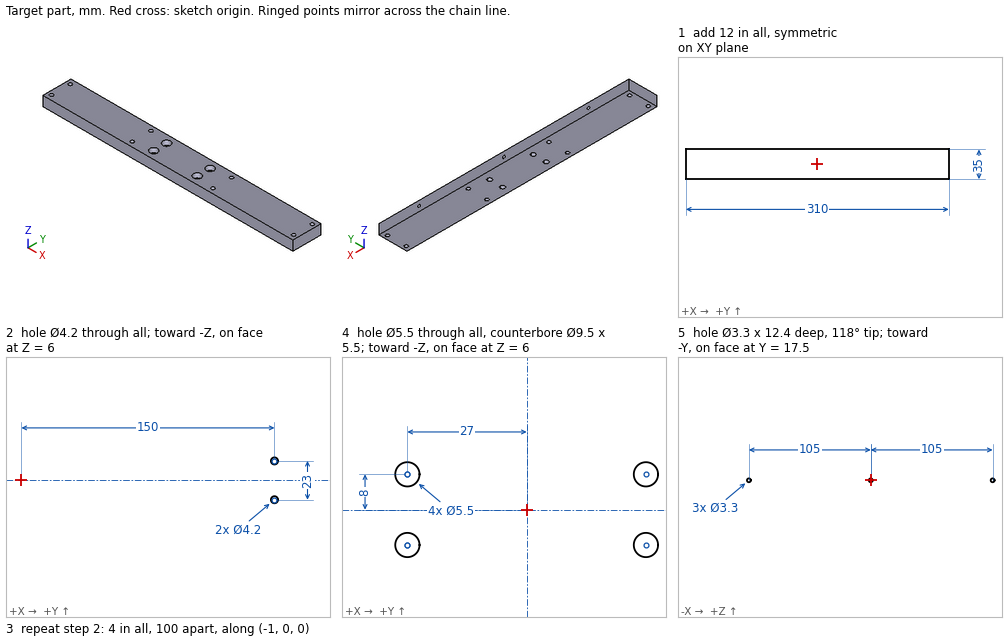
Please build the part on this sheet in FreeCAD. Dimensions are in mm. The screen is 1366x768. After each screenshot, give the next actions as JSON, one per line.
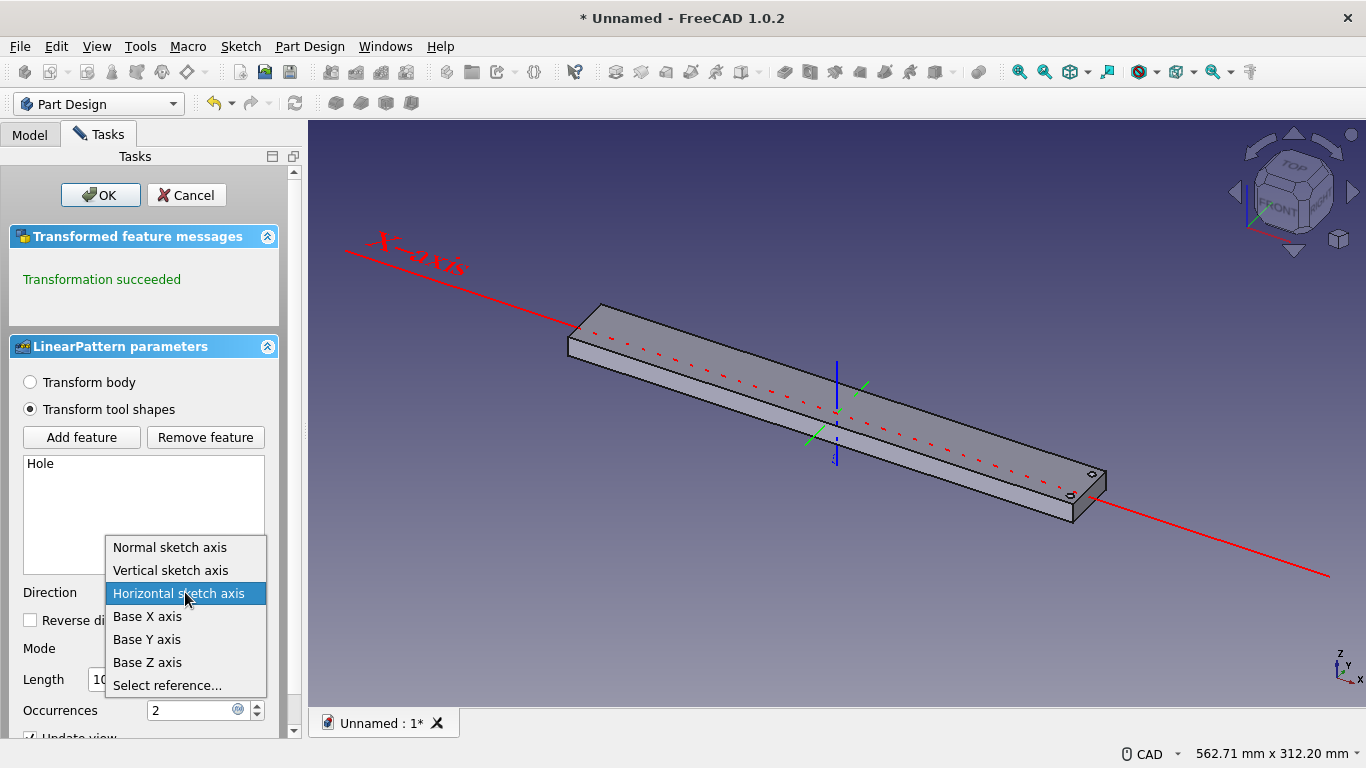
{"action": "left_click", "coordinate": [184, 616]}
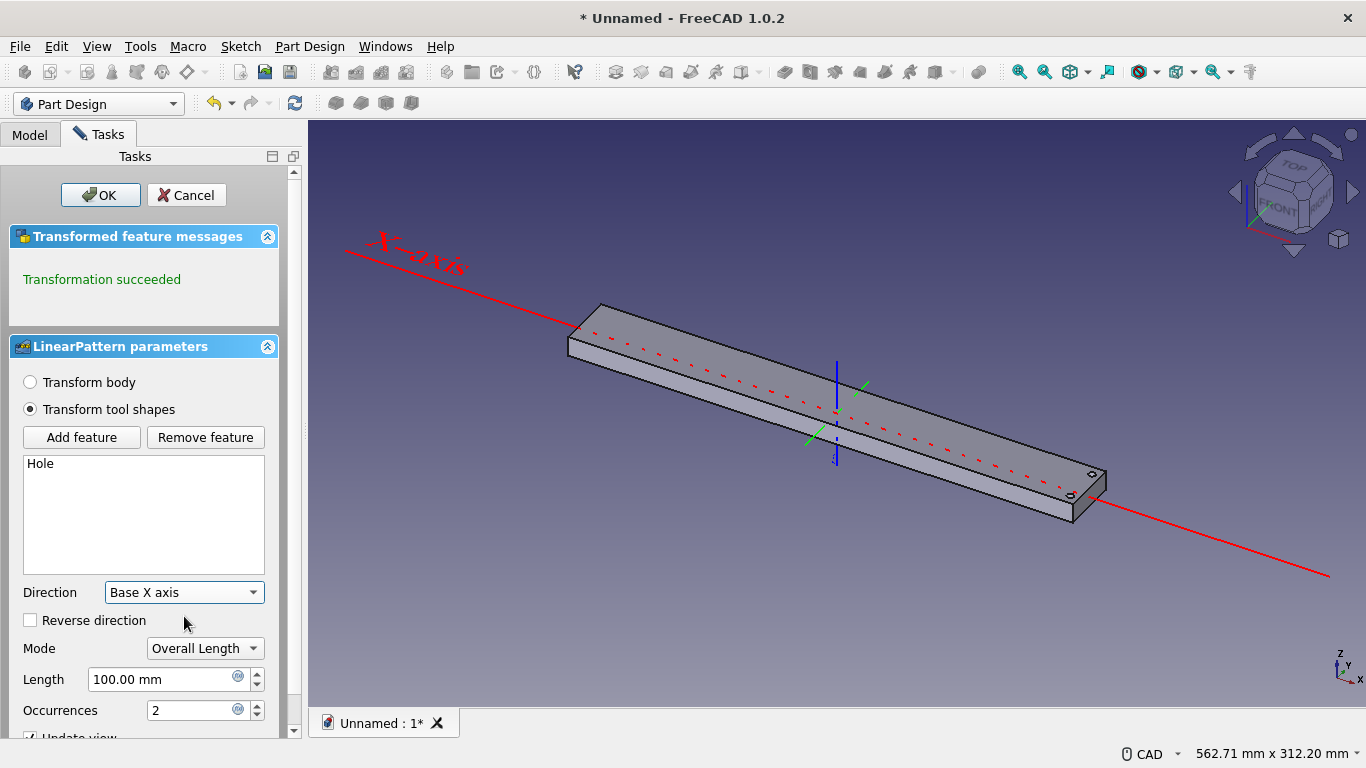
{"action": "left_click", "coordinate": [206, 648]}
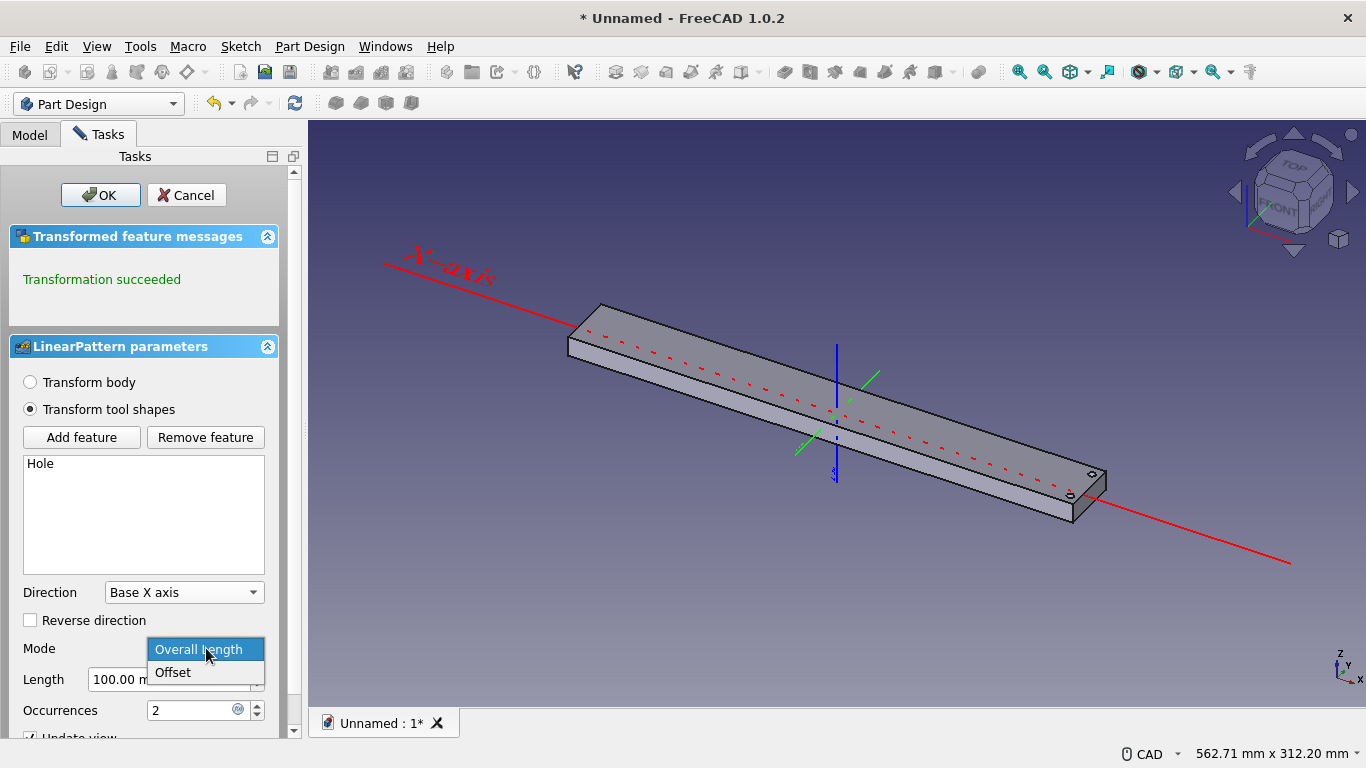
{"action": "left_click", "coordinate": [204, 672]}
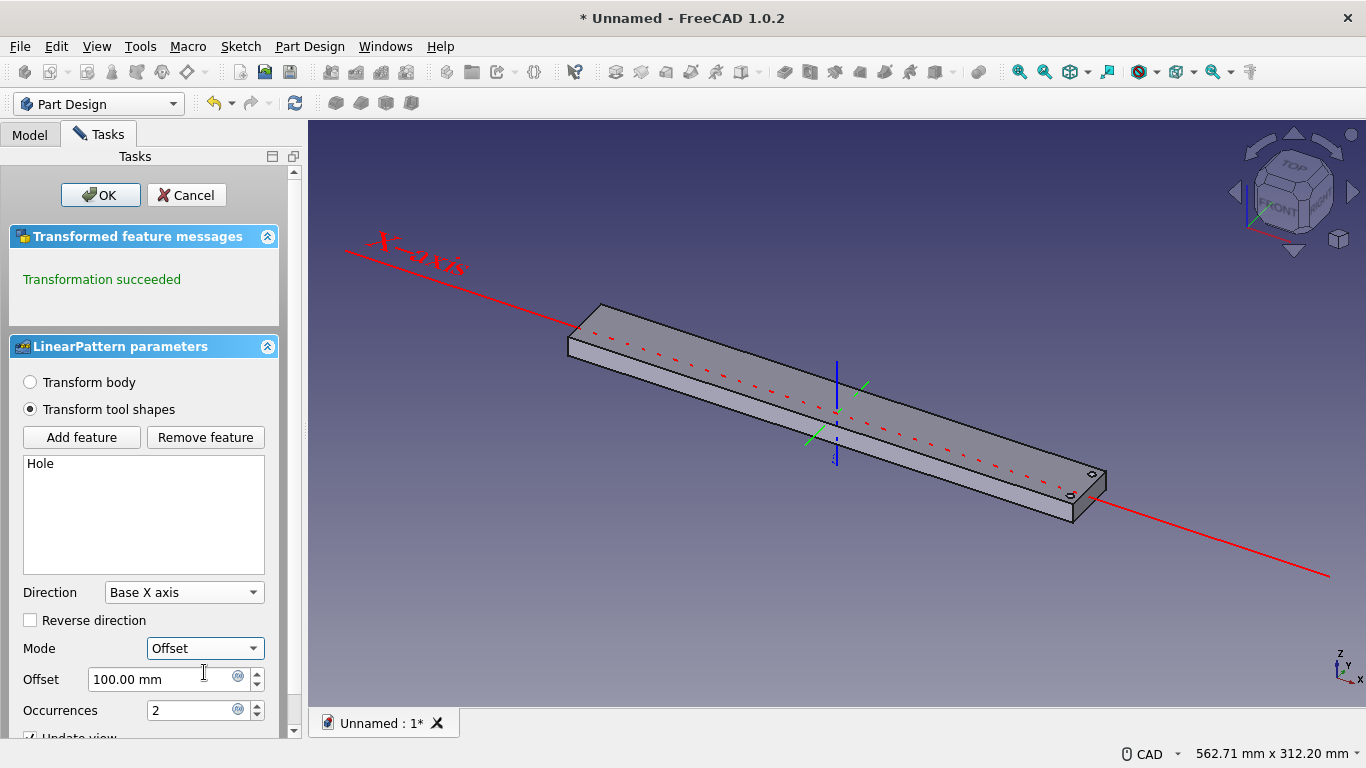
{"action": "triple_click", "coordinate": [170, 680]}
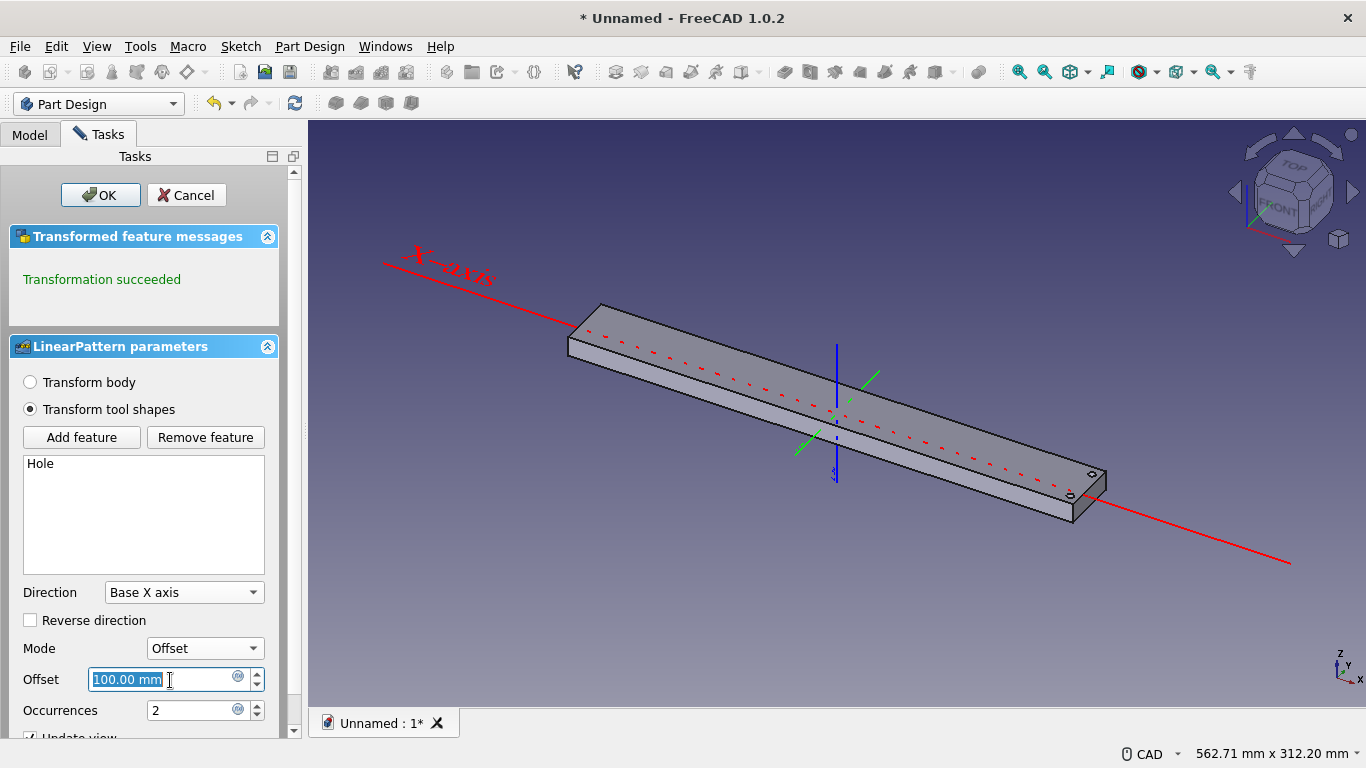
{"action": "type", "text": "100"}
{"action": "key", "text": "Tab"}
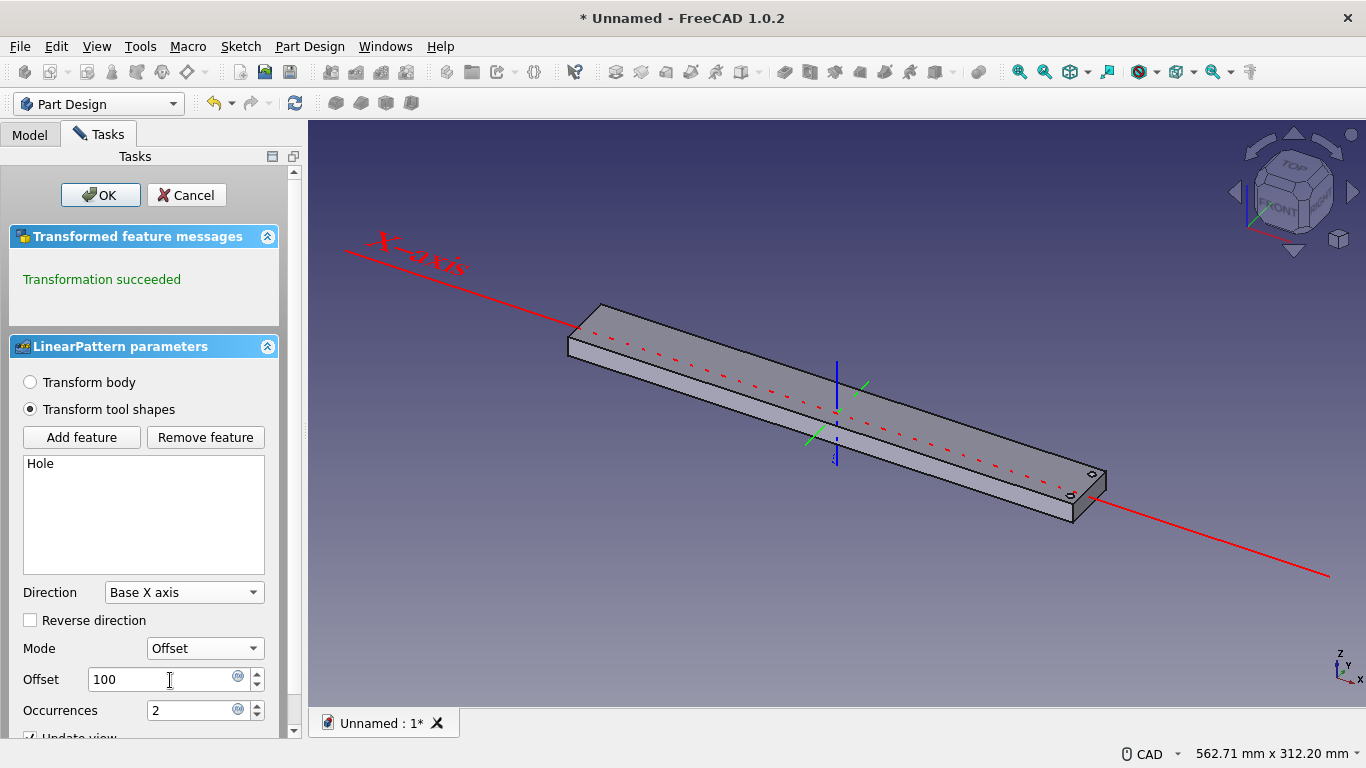
{"action": "triple_click", "coordinate": [199, 710]}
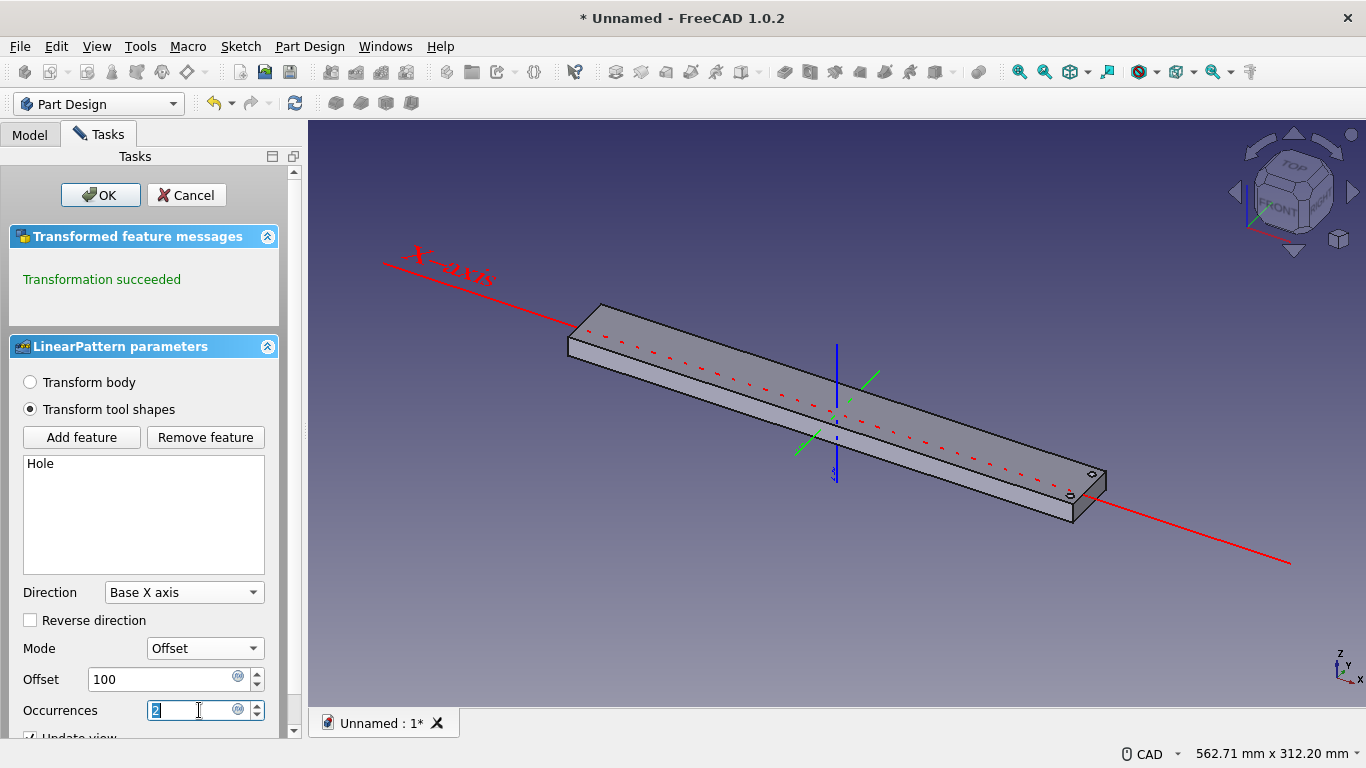
{"action": "type", "text": "4"}
{"action": "key", "text": "Tab"}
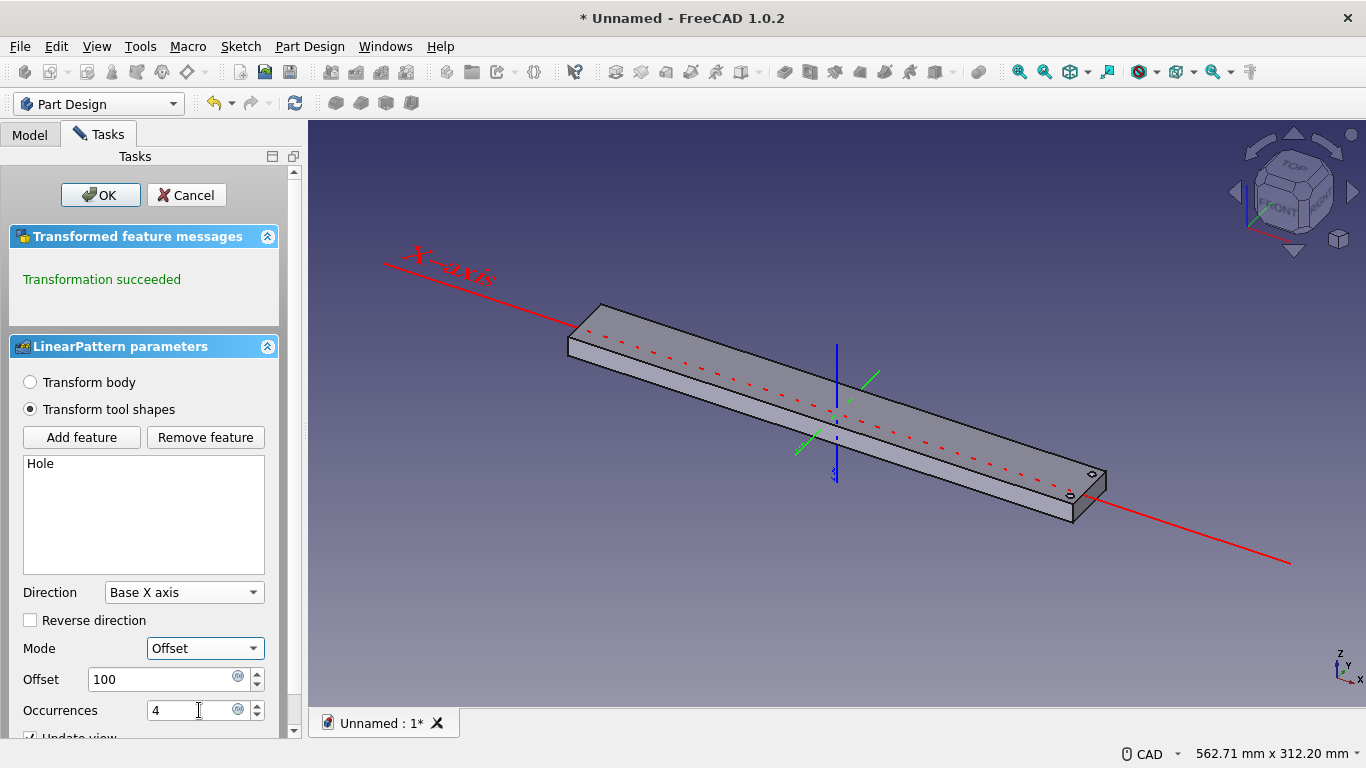
{"action": "left_click", "coordinate": [31, 620]}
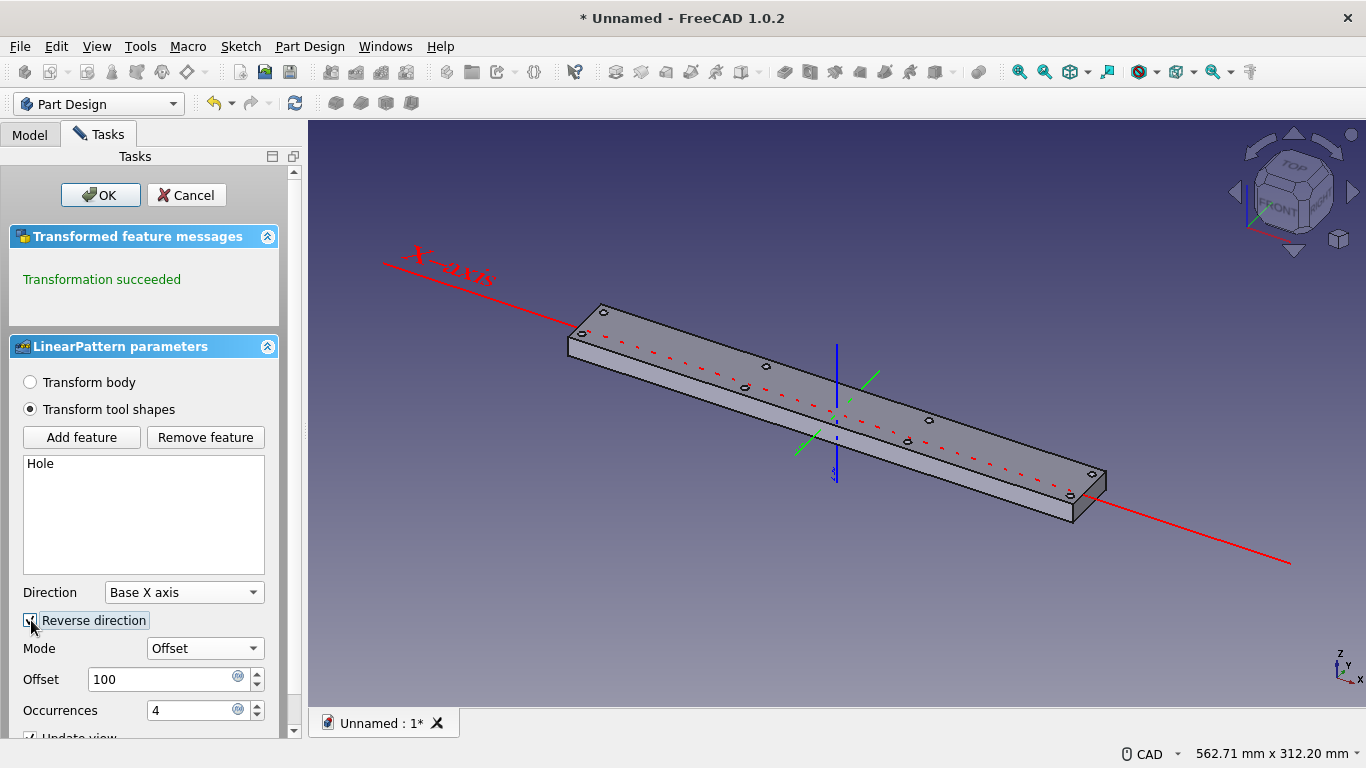
{"action": "left_click", "coordinate": [101, 195]}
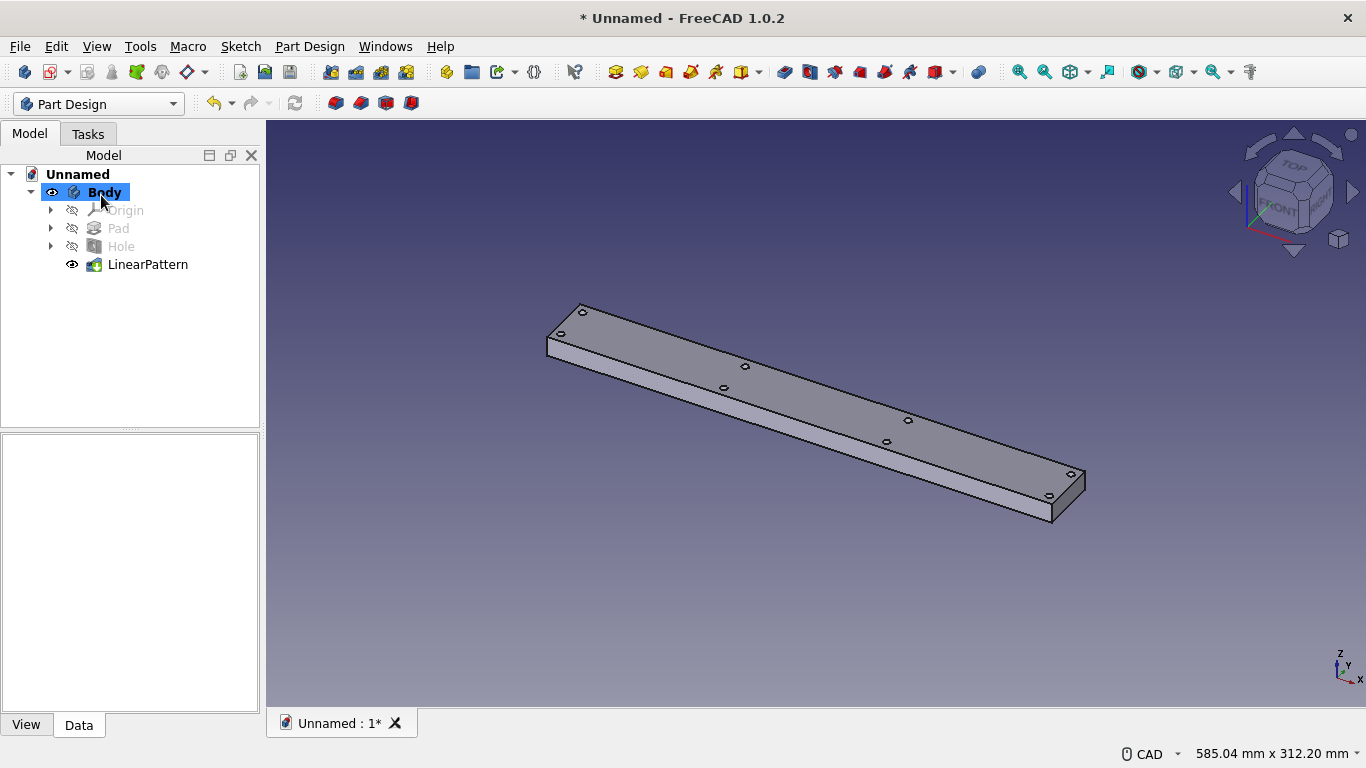
{"action": "left_click", "coordinate": [1032, 475]}